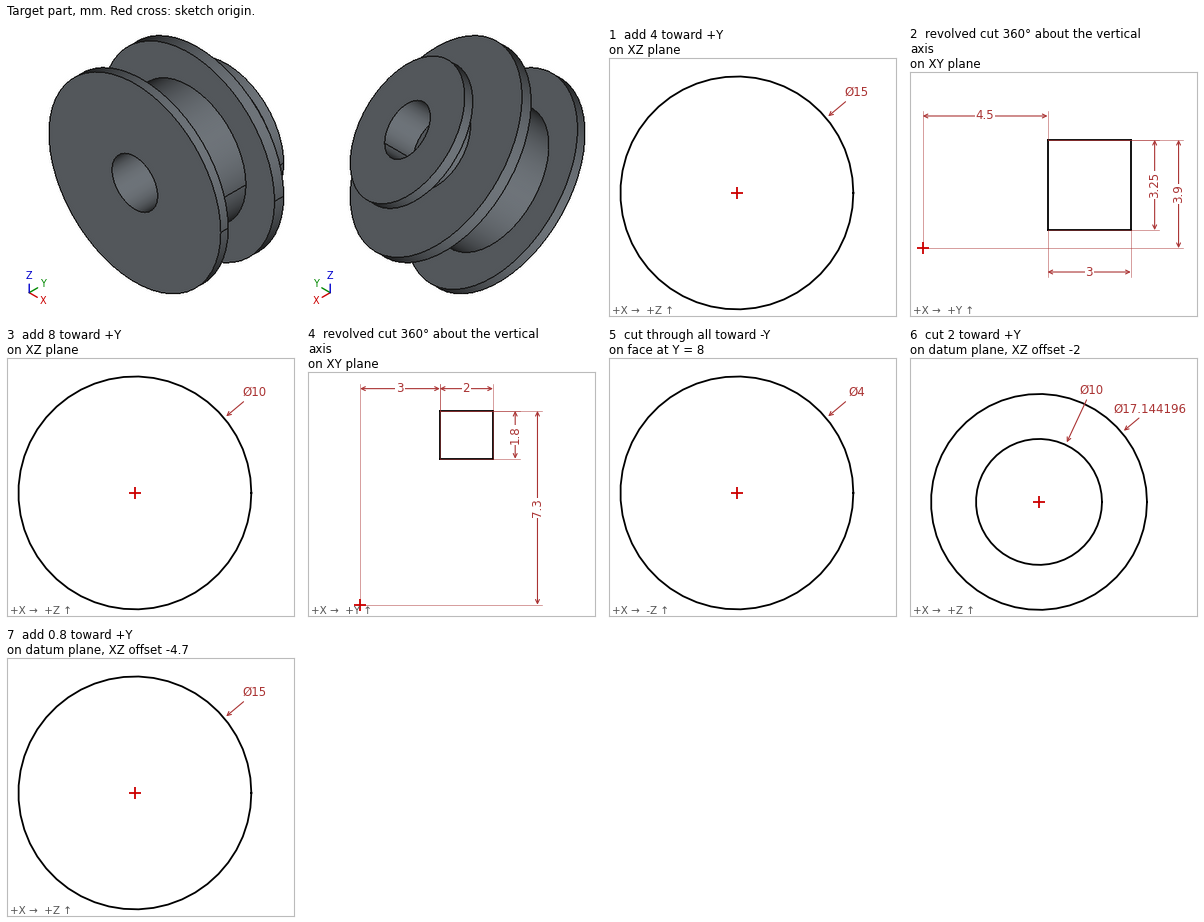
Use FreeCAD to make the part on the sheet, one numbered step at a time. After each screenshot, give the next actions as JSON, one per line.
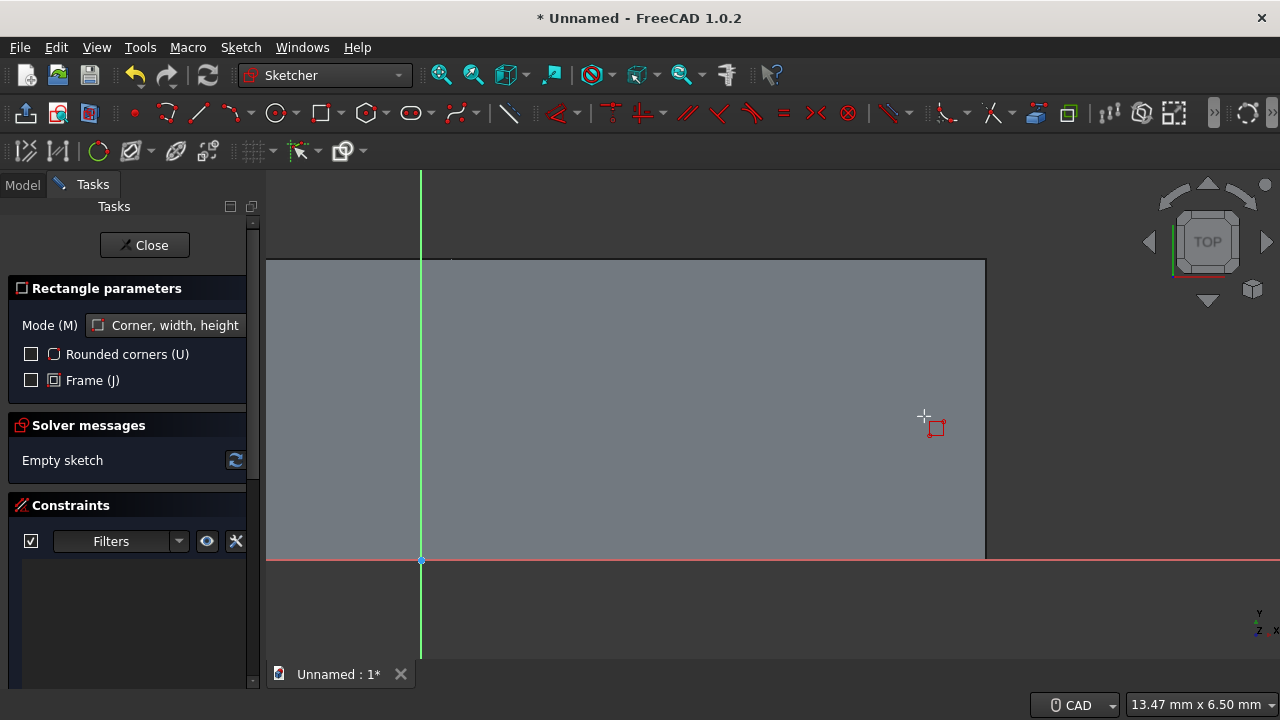
{"action": "left_click", "coordinate": [760, 267]}
{"action": "left_click", "coordinate": [986, 511]}
{"action": "key", "text": "Escape"}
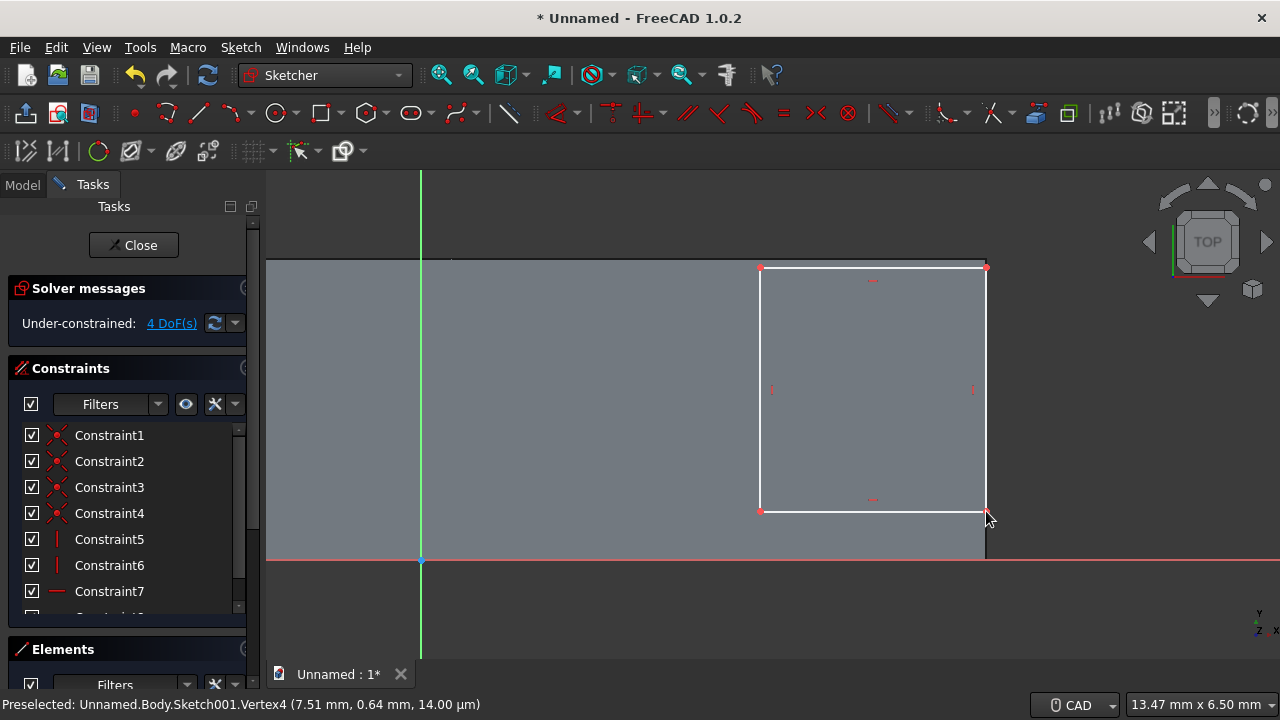
{"action": "left_click", "coordinate": [556, 114]}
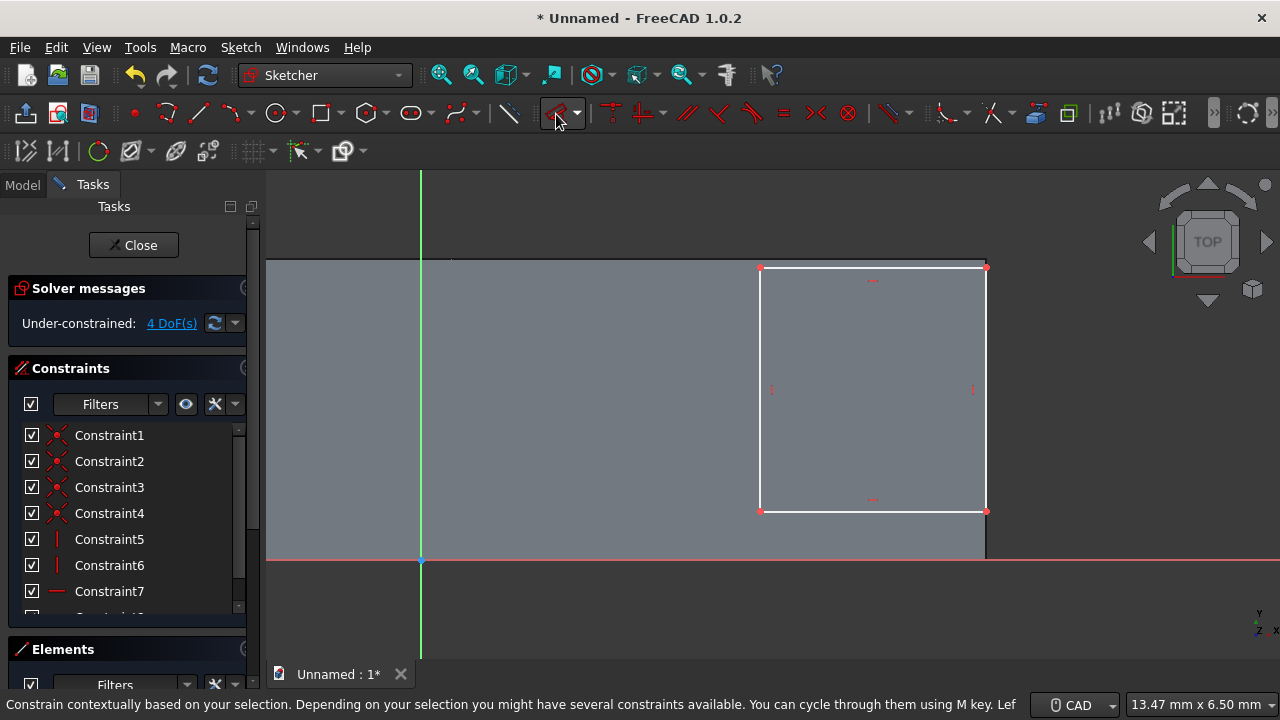
{"action": "left_click", "coordinate": [828, 512]}
{"action": "left_click", "coordinate": [873, 546]}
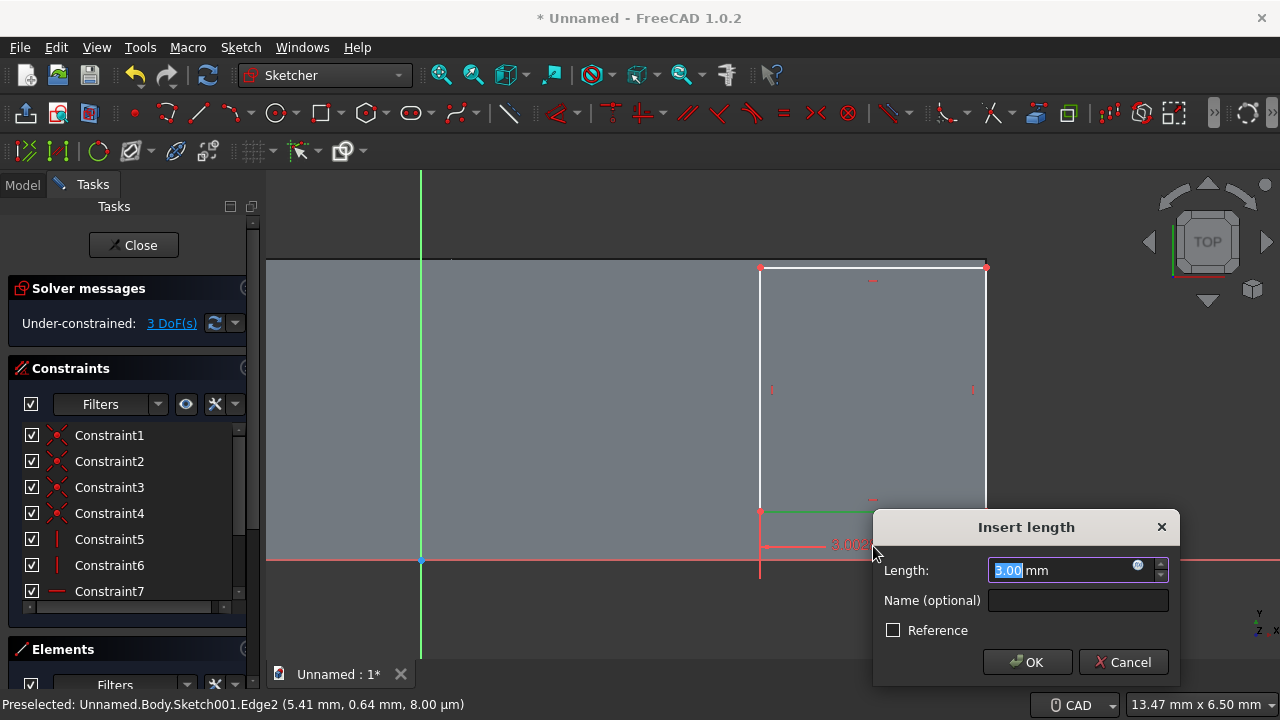
{"action": "type", "text": "3"}
{"action": "key", "text": "Return"}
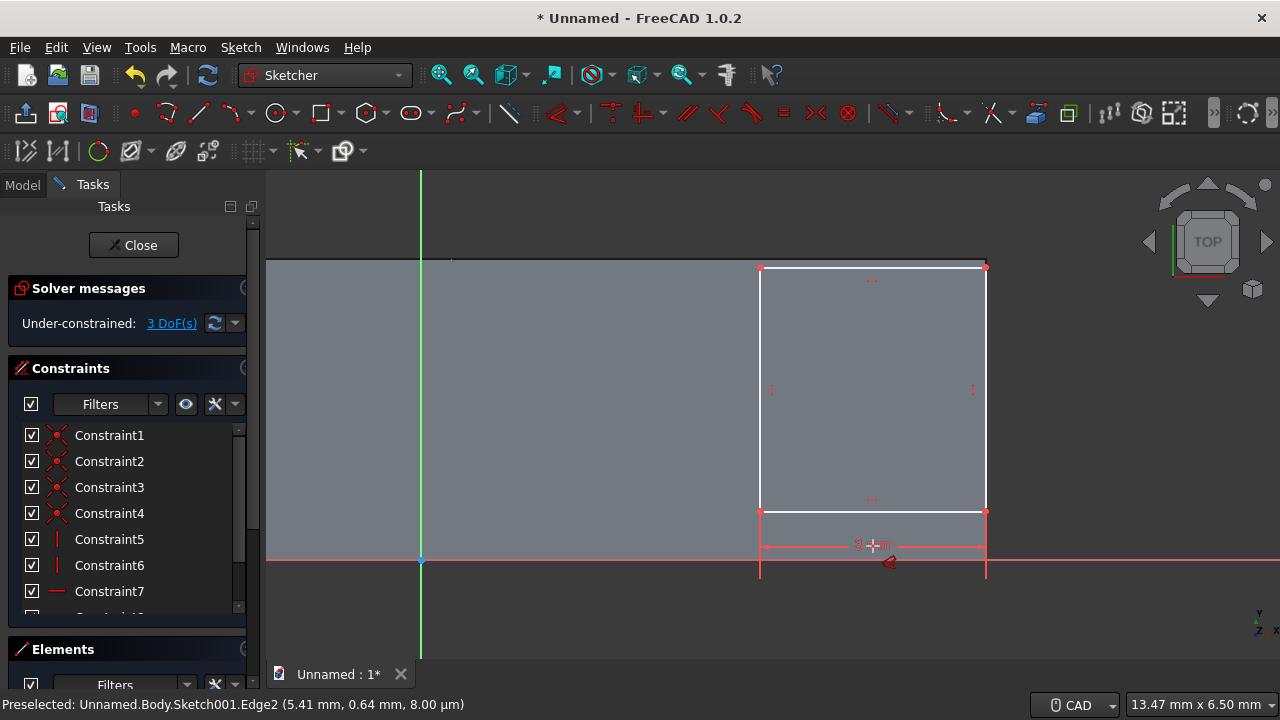
{"action": "left_click", "coordinate": [760, 341]}
{"action": "left_click", "coordinate": [794, 390]}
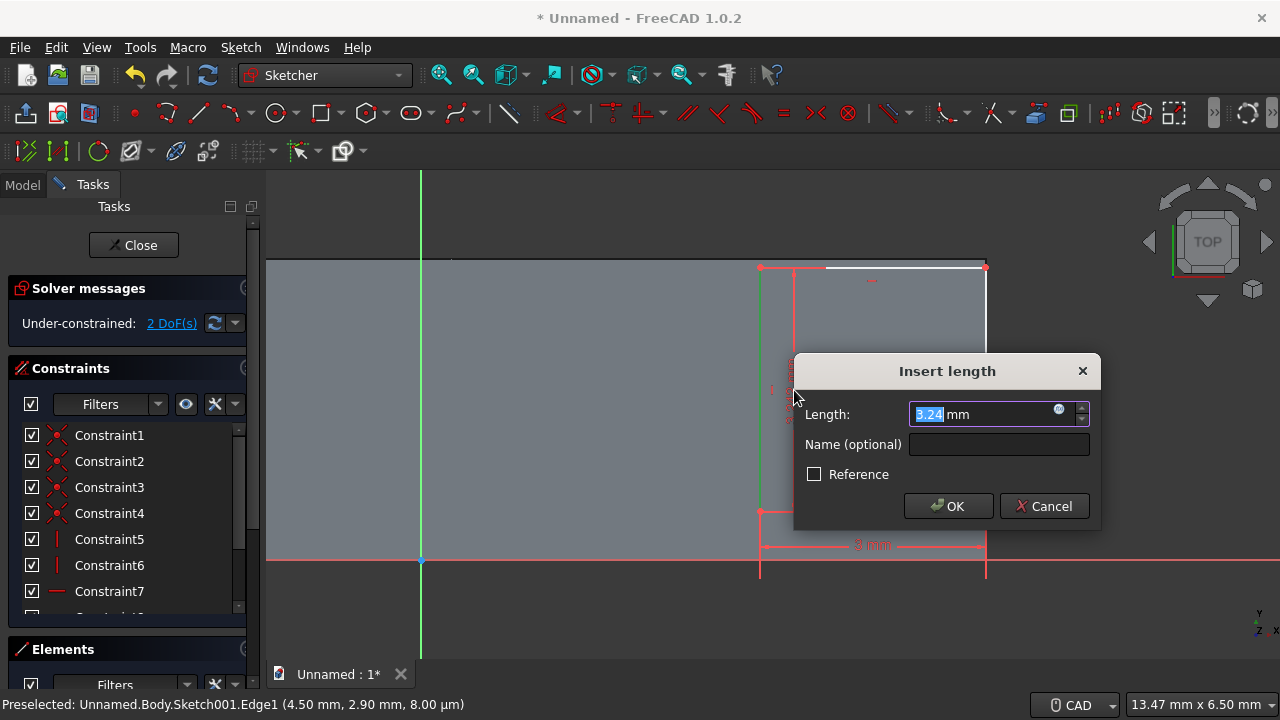
{"action": "type", "text": "3.25"}
{"action": "key", "text": "Return"}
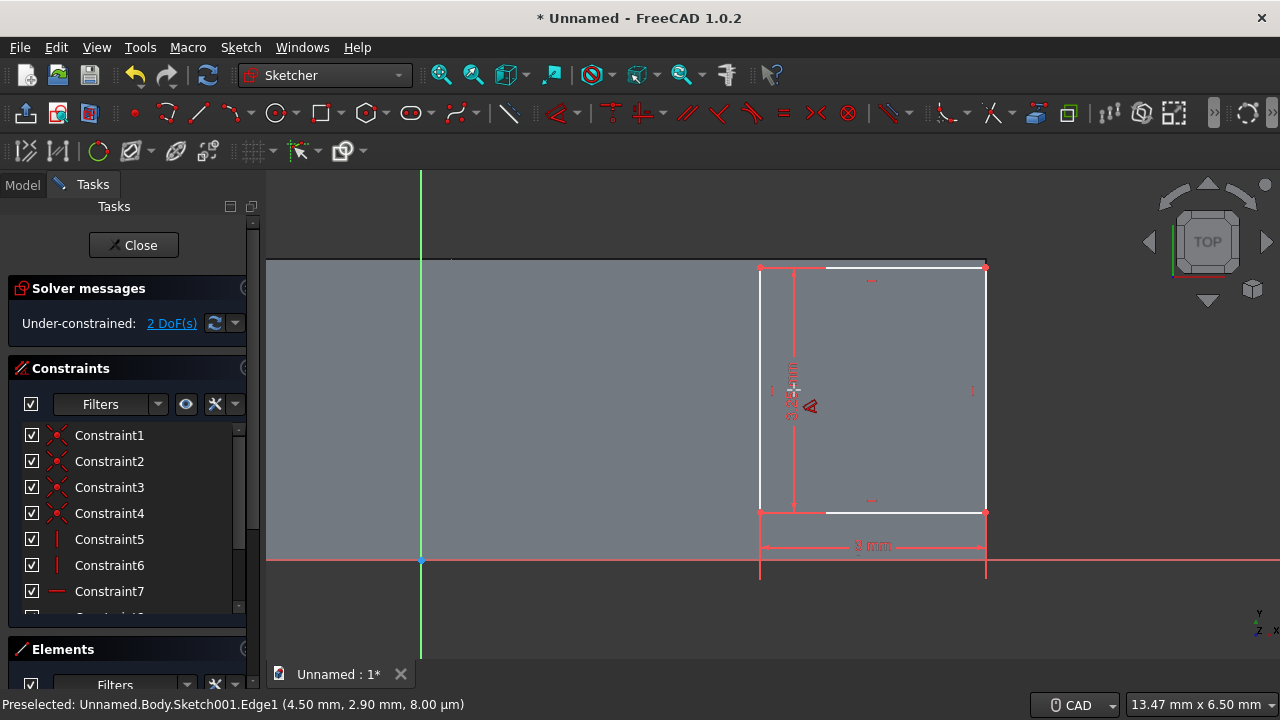
{"action": "left_click", "coordinate": [760, 268]}
{"action": "left_click", "coordinate": [591, 594]}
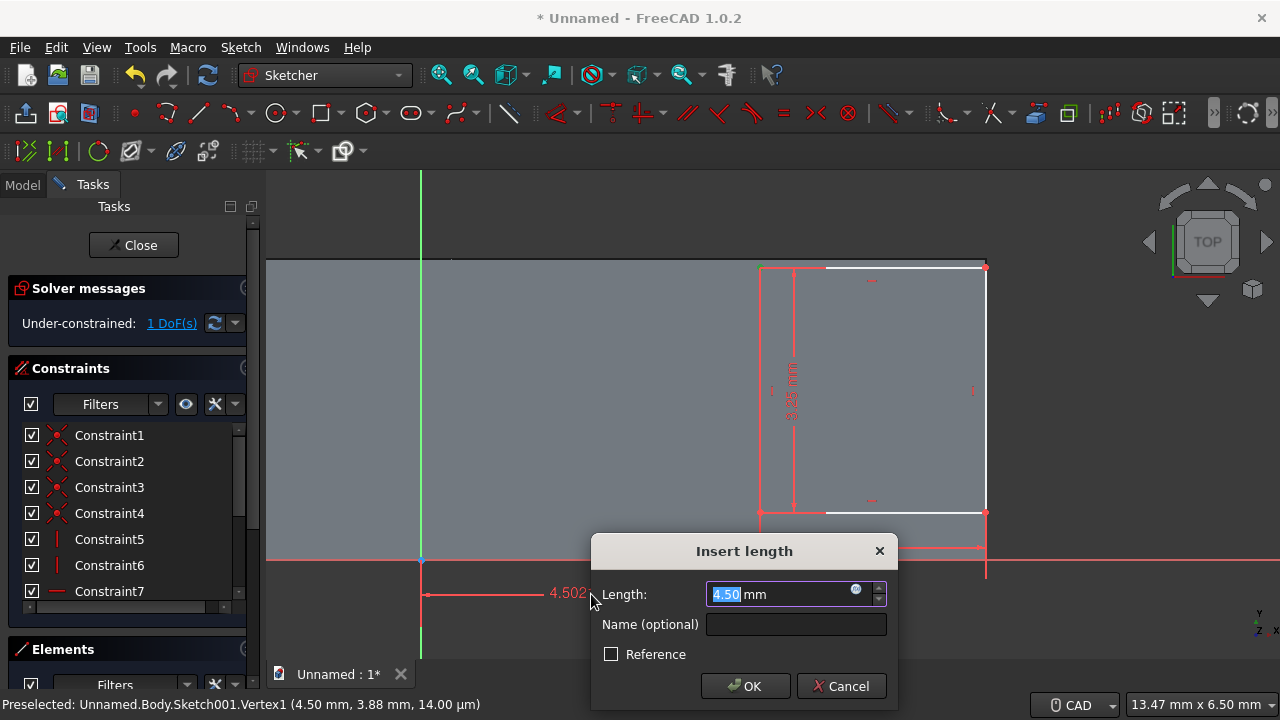
{"action": "type", "text": "4.5"}
{"action": "key", "text": "Return"}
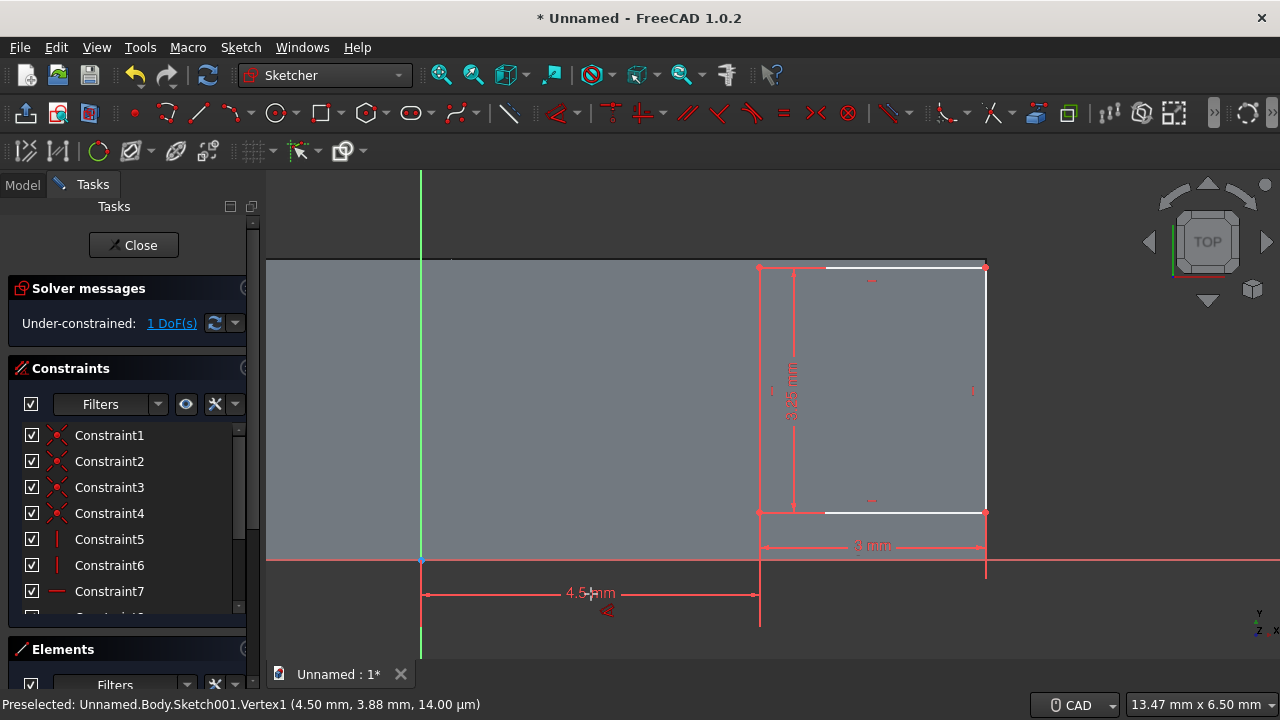
{"action": "left_click", "coordinate": [760, 268]}
{"action": "left_click", "coordinate": [387, 414]}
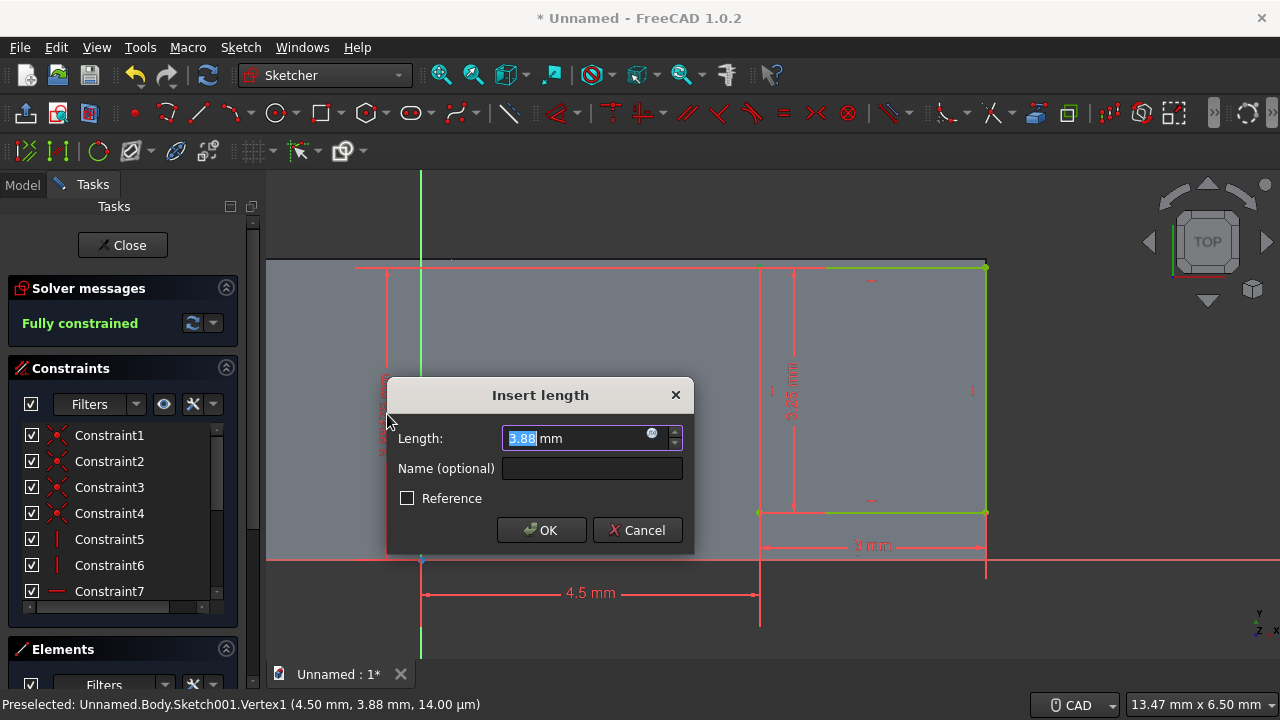
{"action": "type", "text": "3.9"}
{"action": "key", "text": "Return"}
{"action": "key", "text": "Escape"}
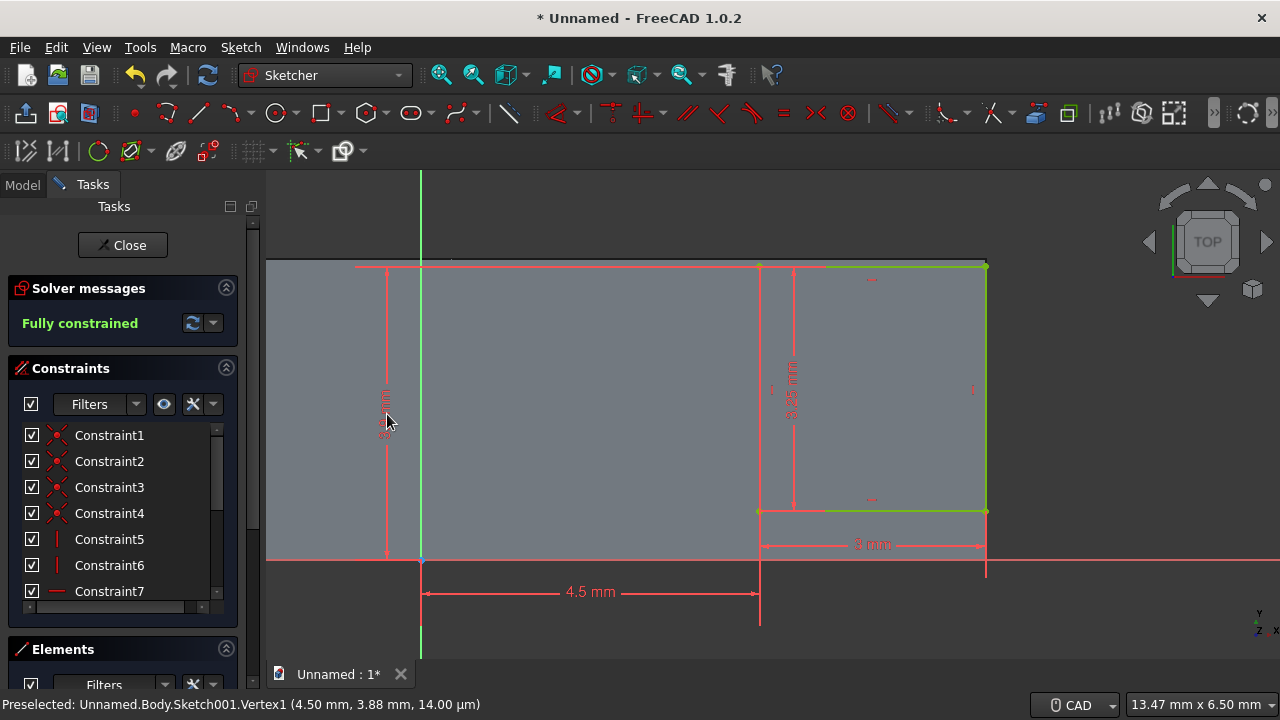
{"action": "left_click", "coordinate": [123, 245]}